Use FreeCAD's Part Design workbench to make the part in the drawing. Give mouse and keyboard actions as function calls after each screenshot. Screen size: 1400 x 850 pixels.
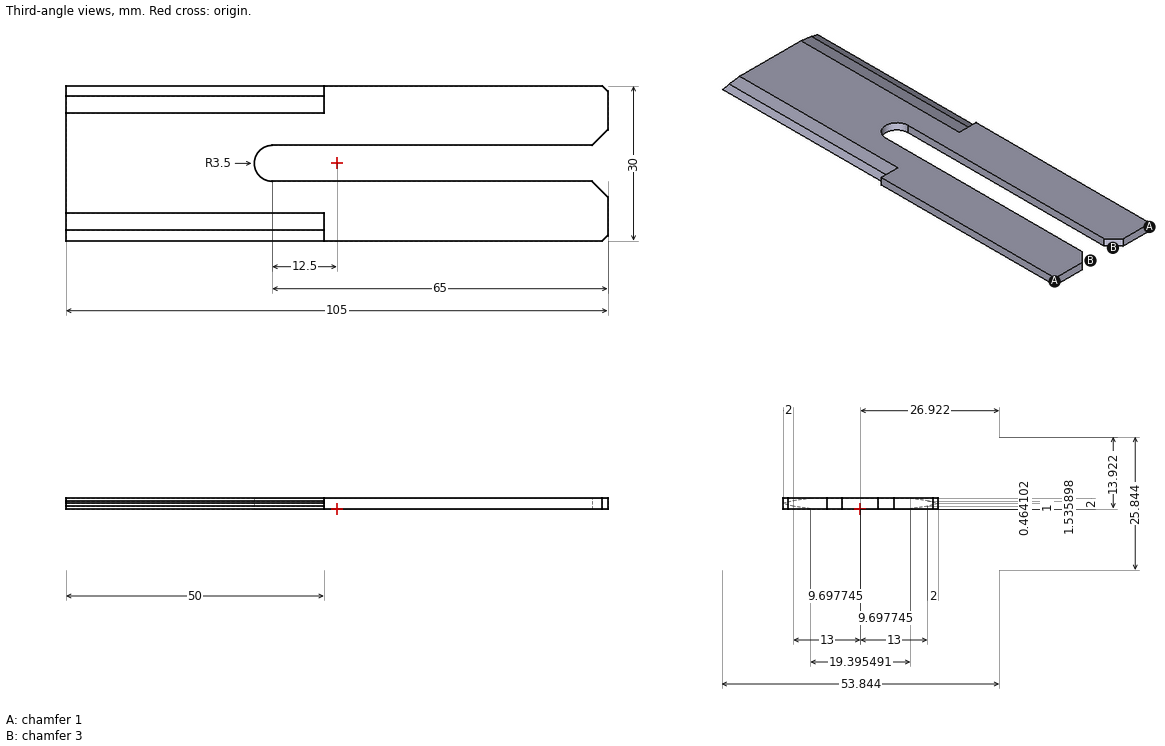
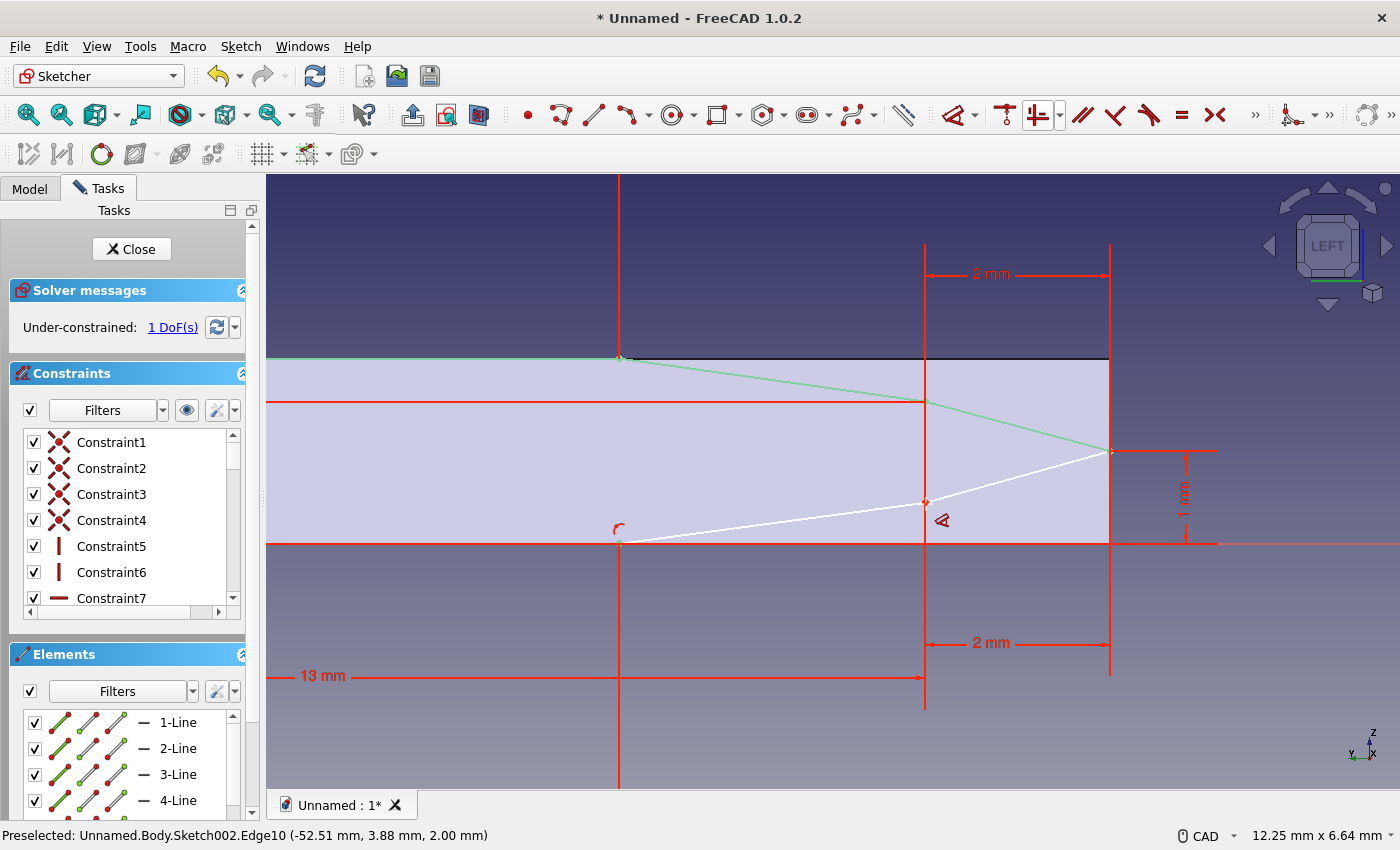
click(925, 503)
click(959, 523)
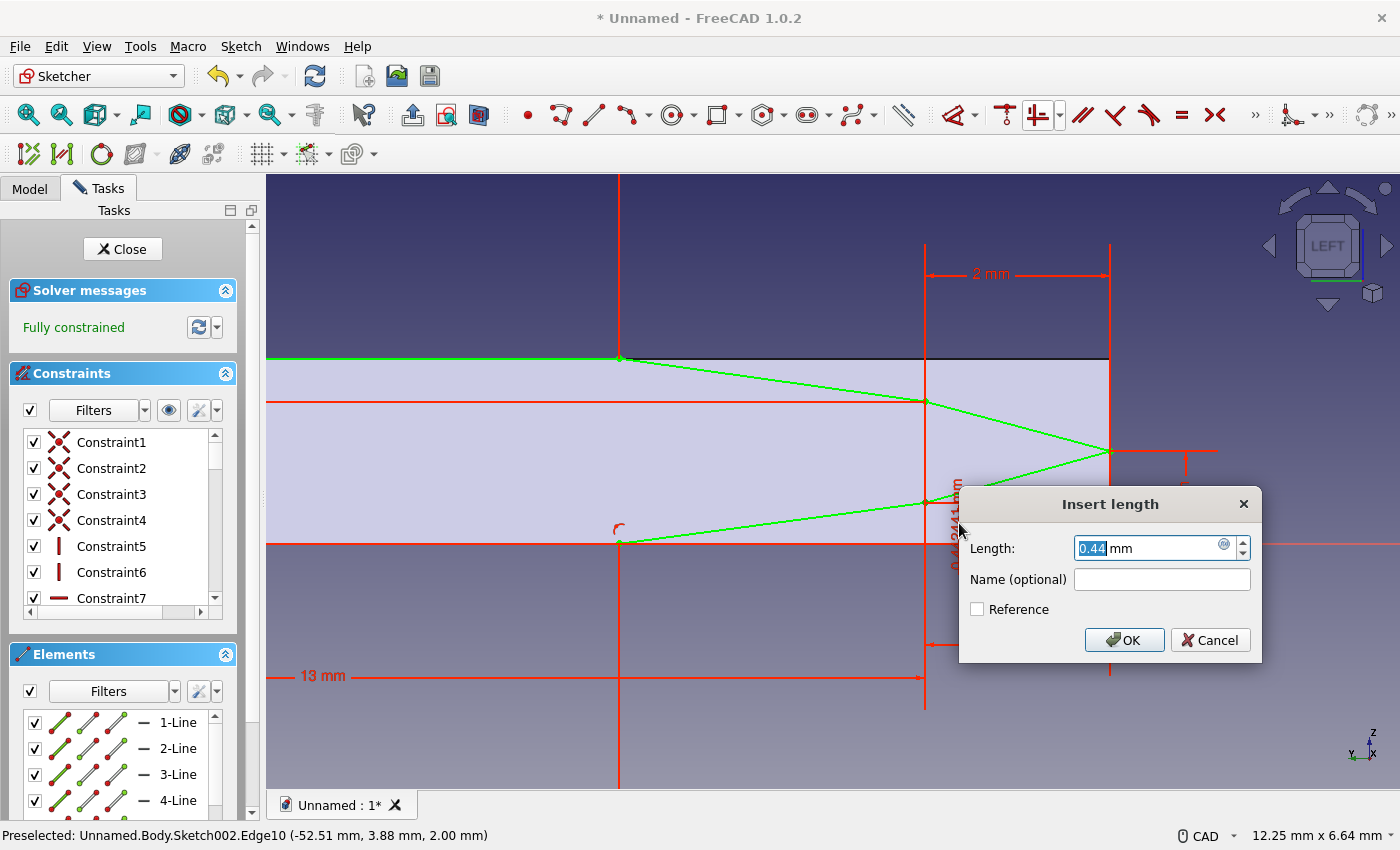
text(0.464102)
key(Return)
key(Escape)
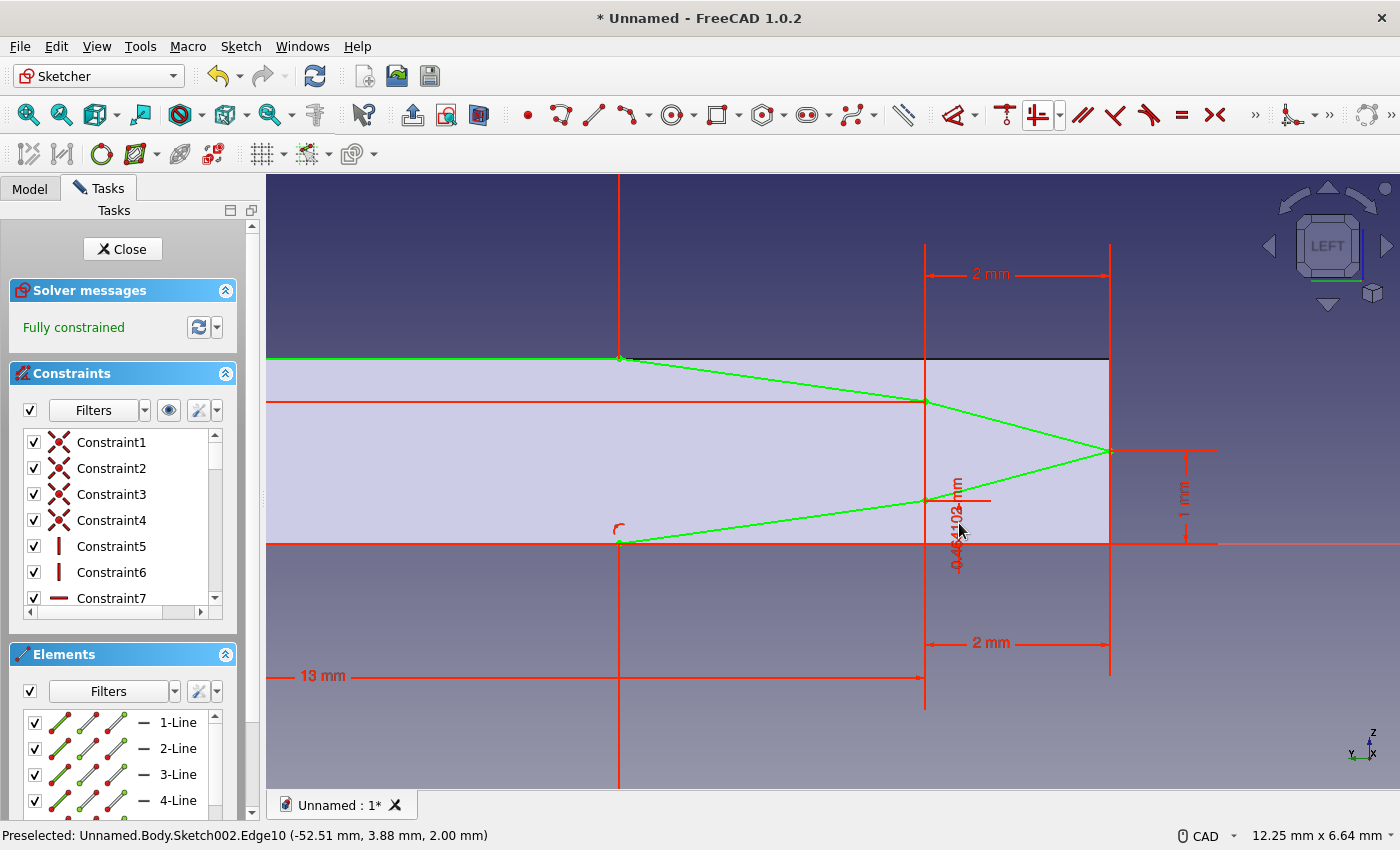
click(123, 249)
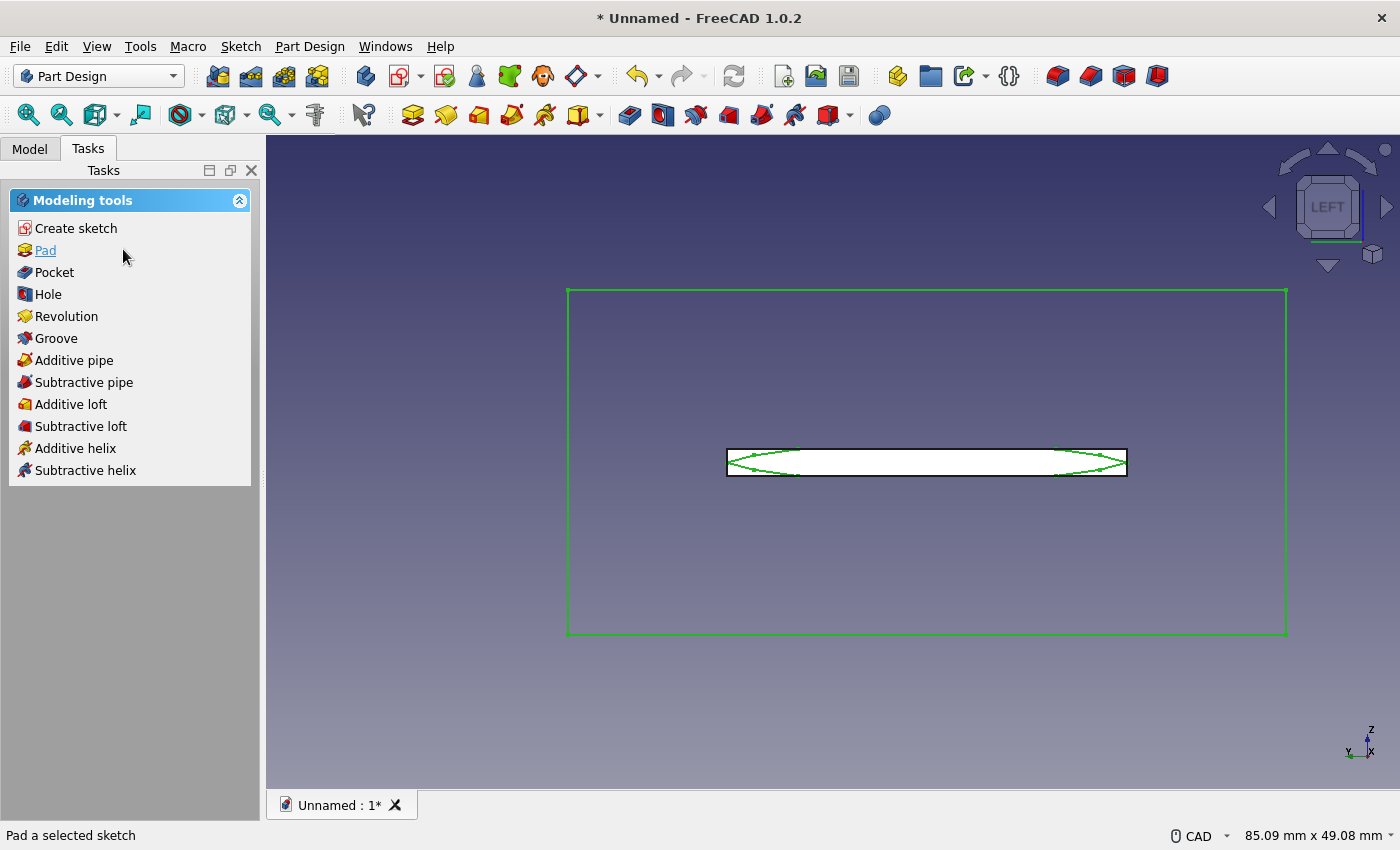
click(630, 116)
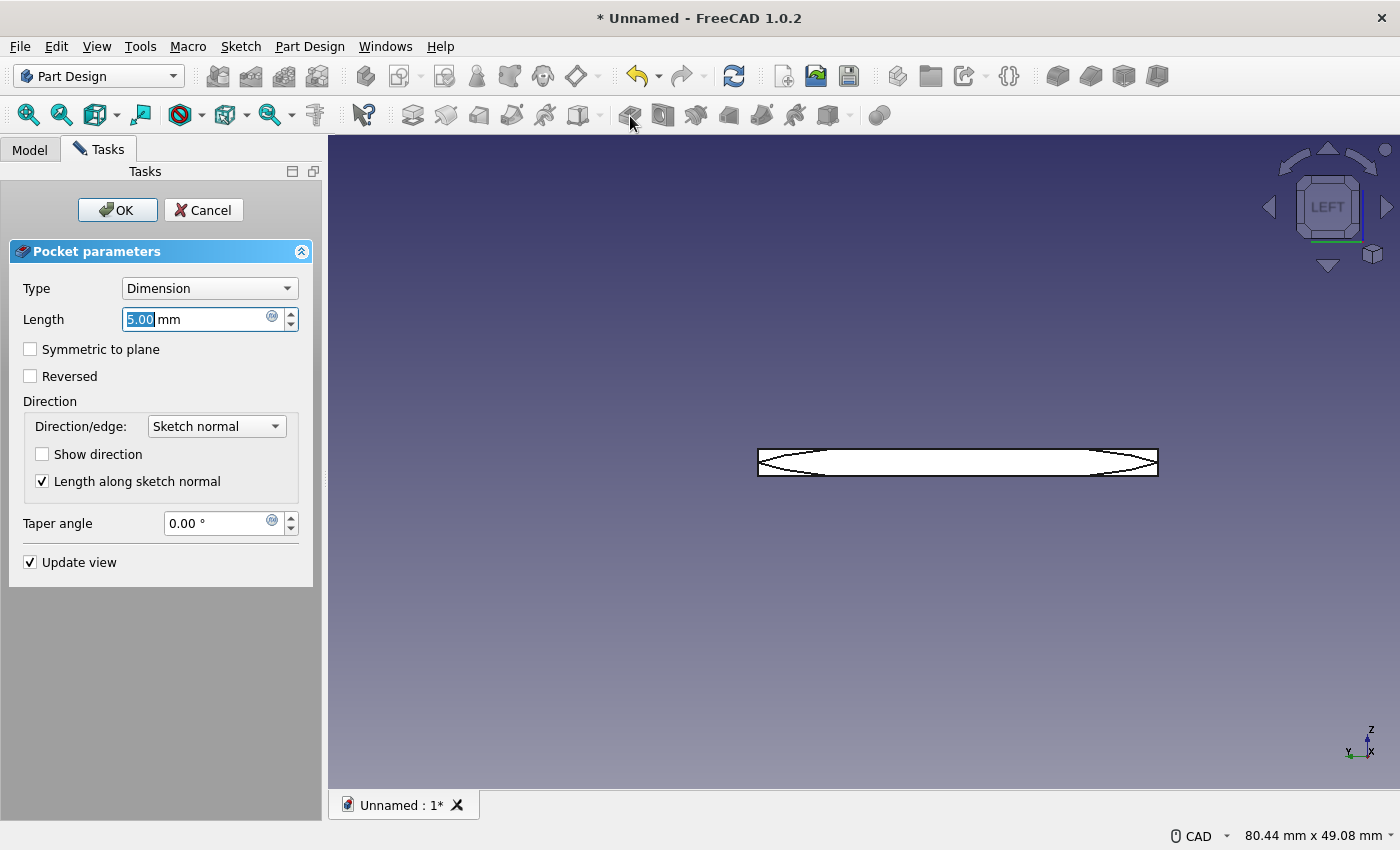
text(50)
key(Tab)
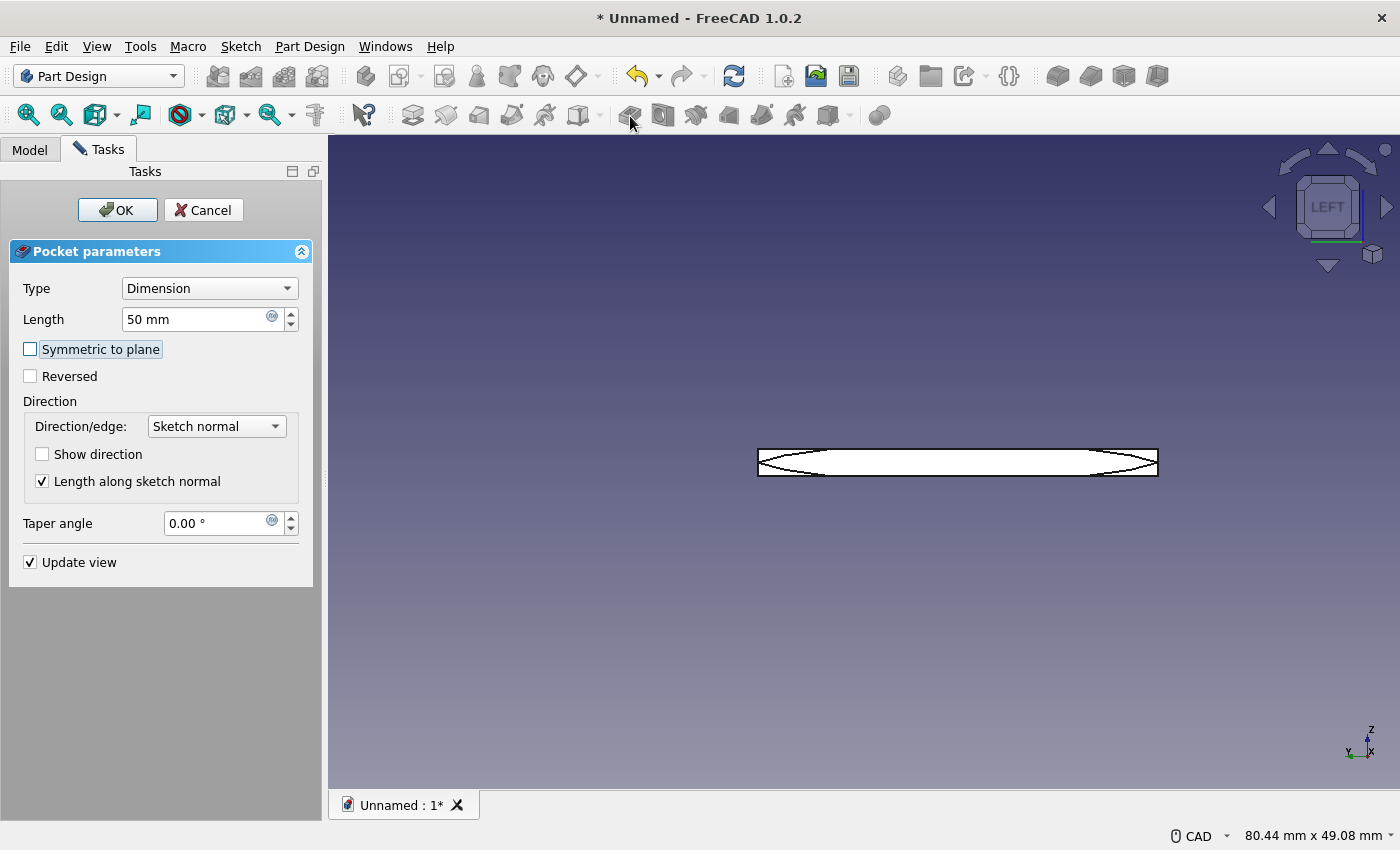
click(118, 210)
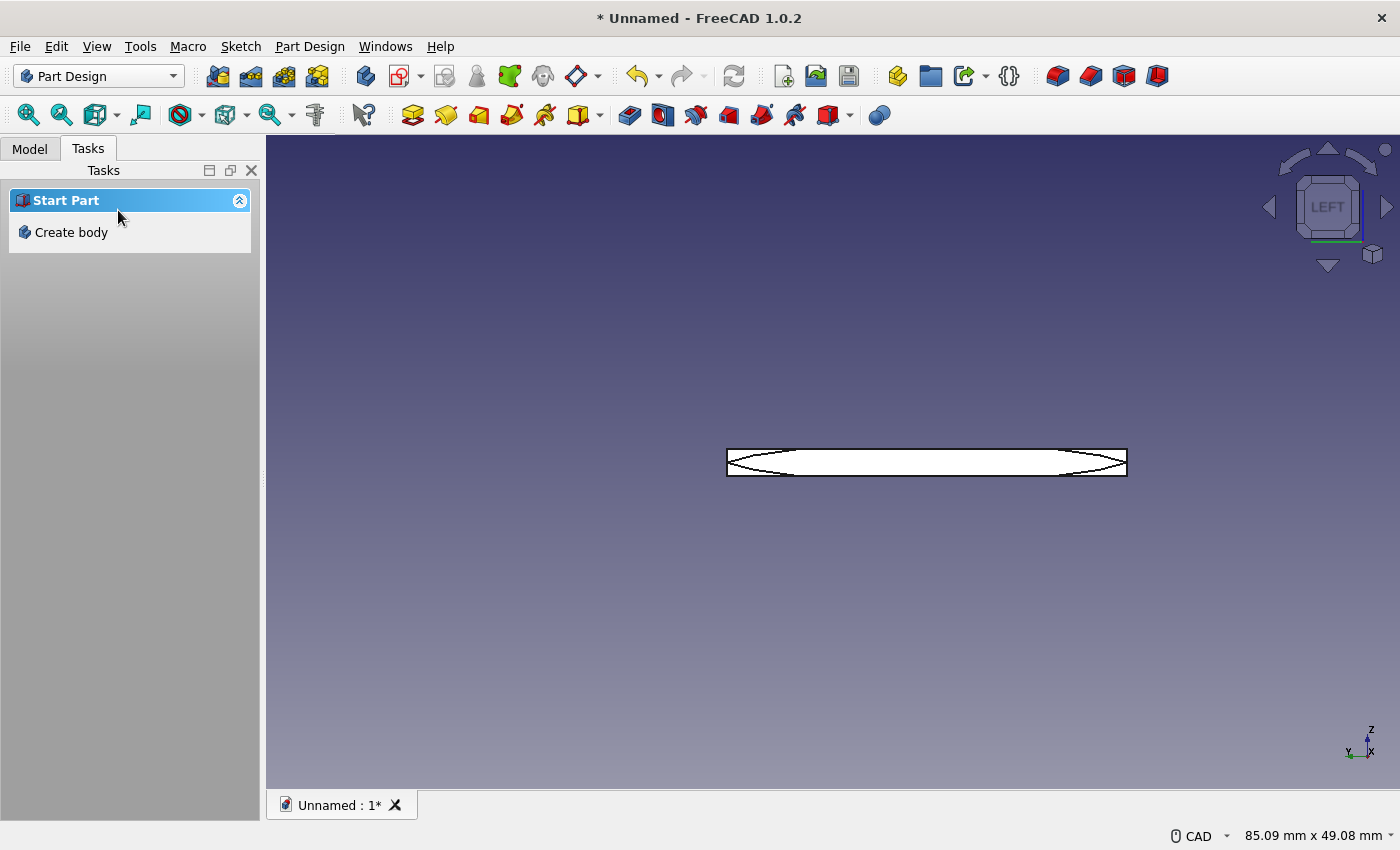
click(29, 116)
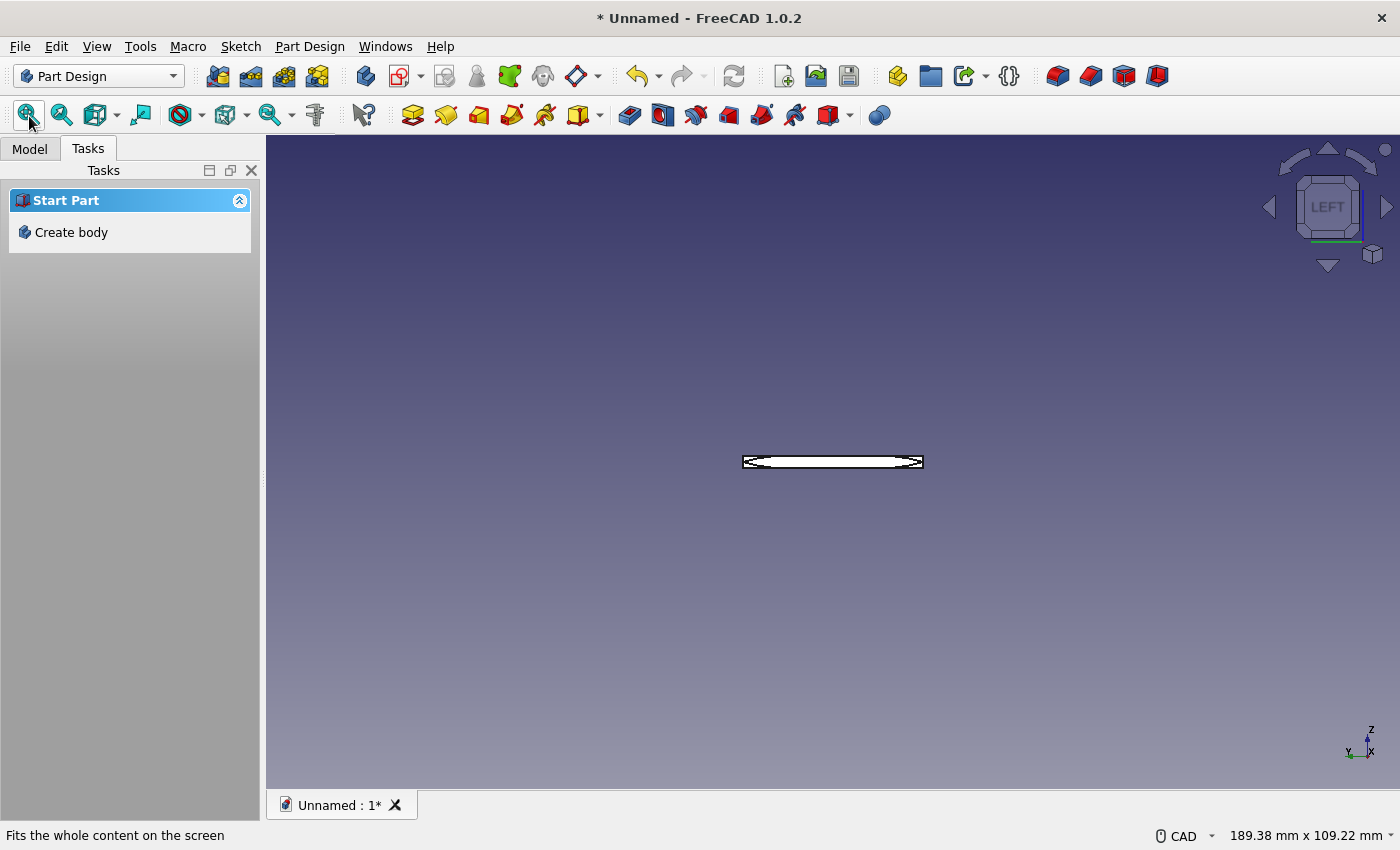
scroll(923, 461, up, 7)